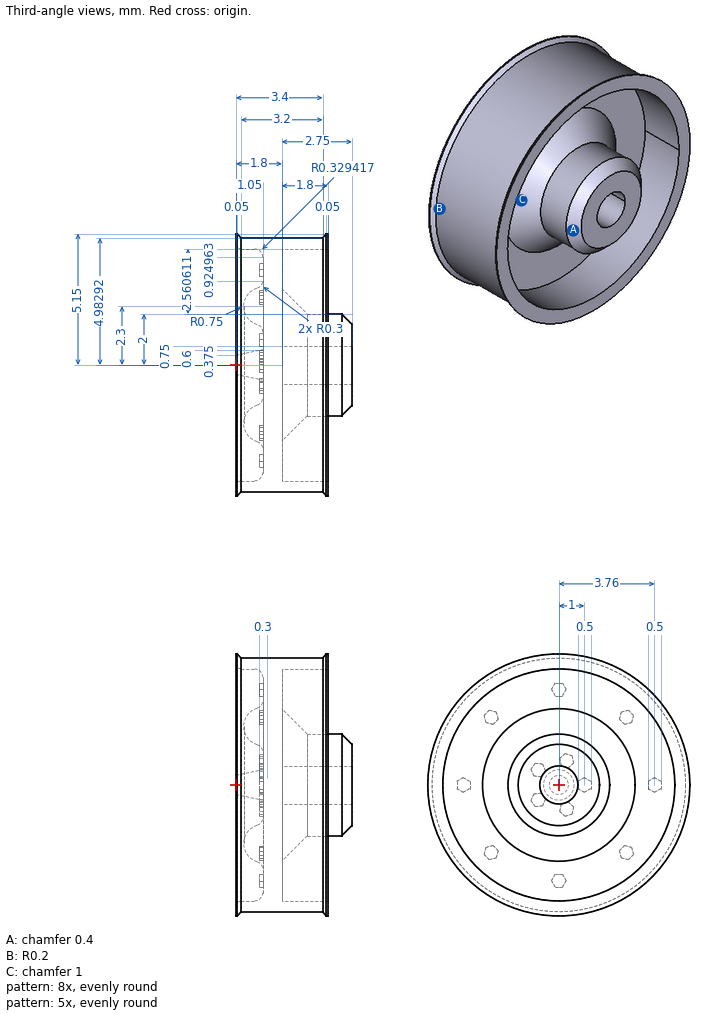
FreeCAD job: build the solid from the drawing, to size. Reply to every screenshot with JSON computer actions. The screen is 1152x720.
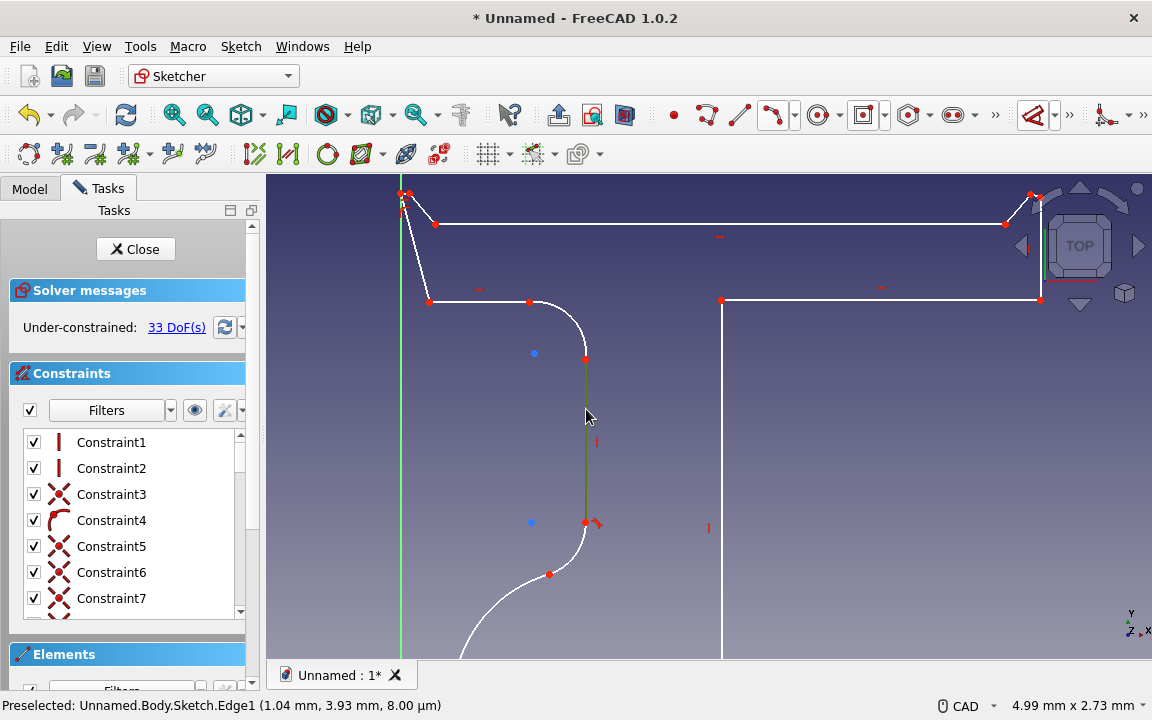
{"action": "left_click", "coordinate": [582, 333]}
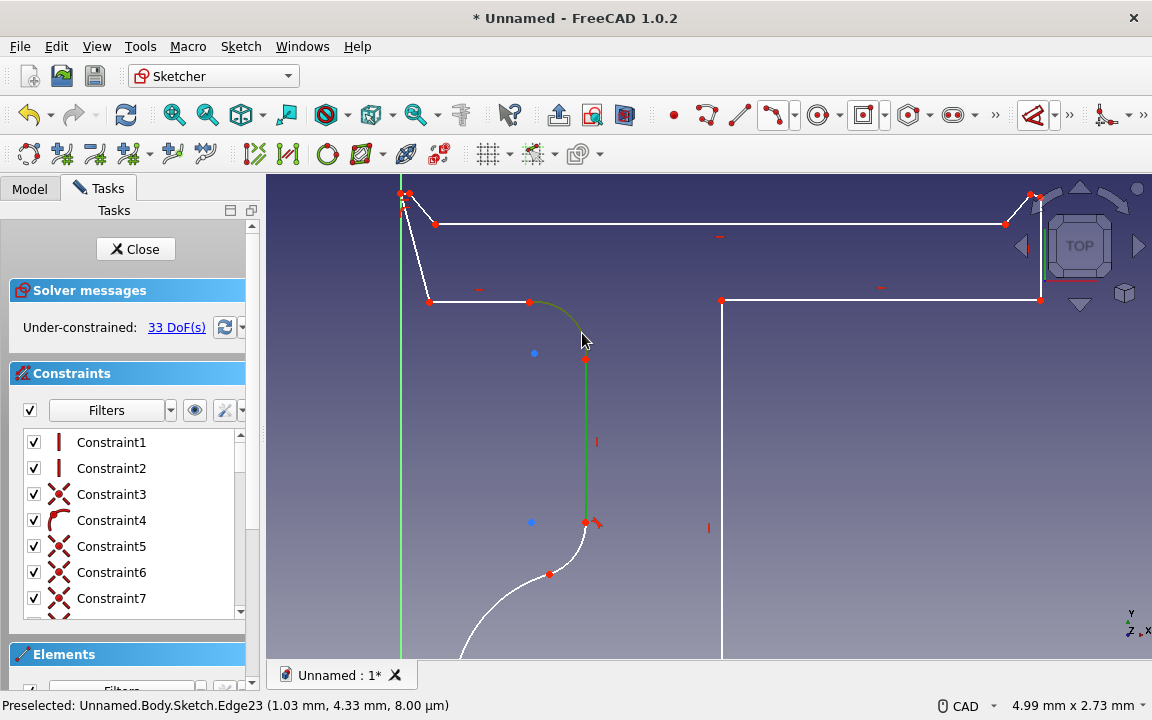
{"action": "key", "text": "t"}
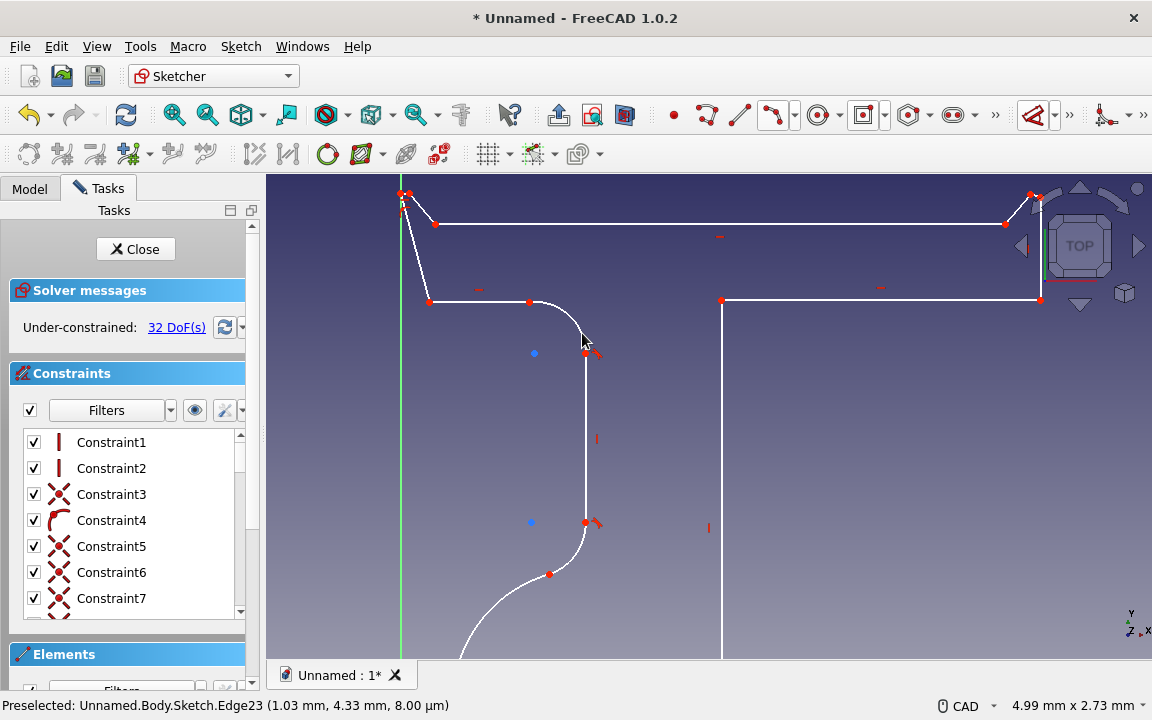
{"action": "scroll", "coordinate": [570, 316], "scroll_direction": "down", "scroll_amount": 6}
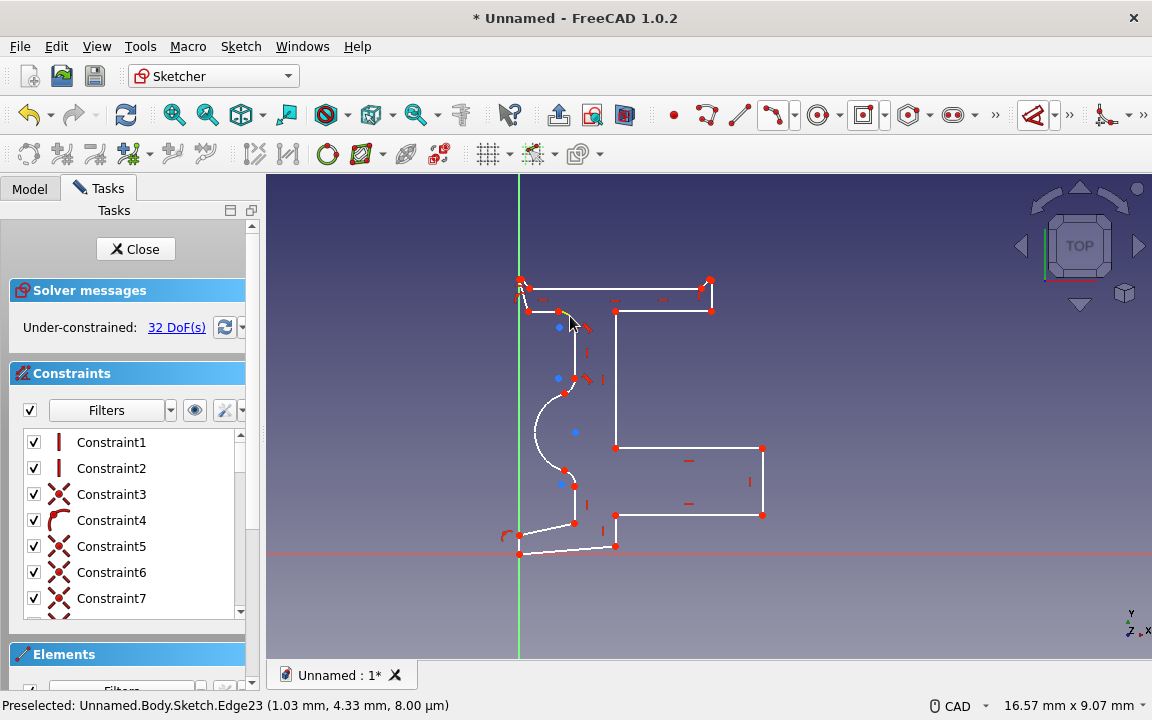
{"action": "scroll", "coordinate": [575, 498], "scroll_direction": "up", "scroll_amount": 2}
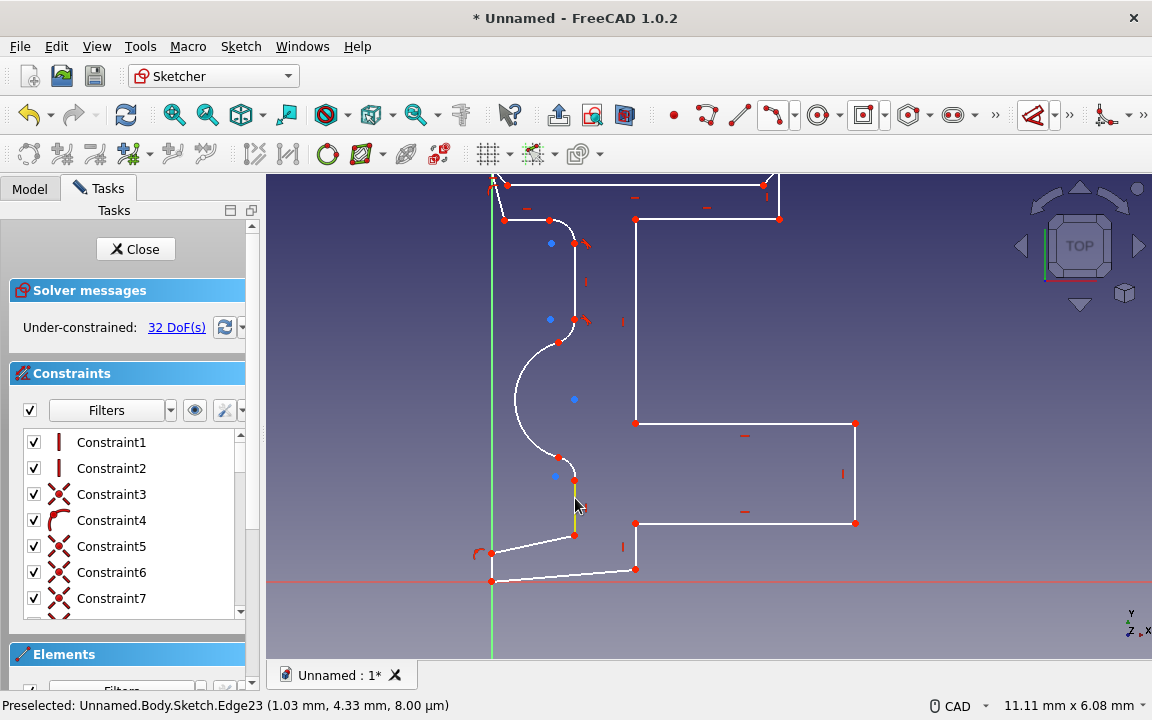
{"action": "left_click", "coordinate": [575, 497]}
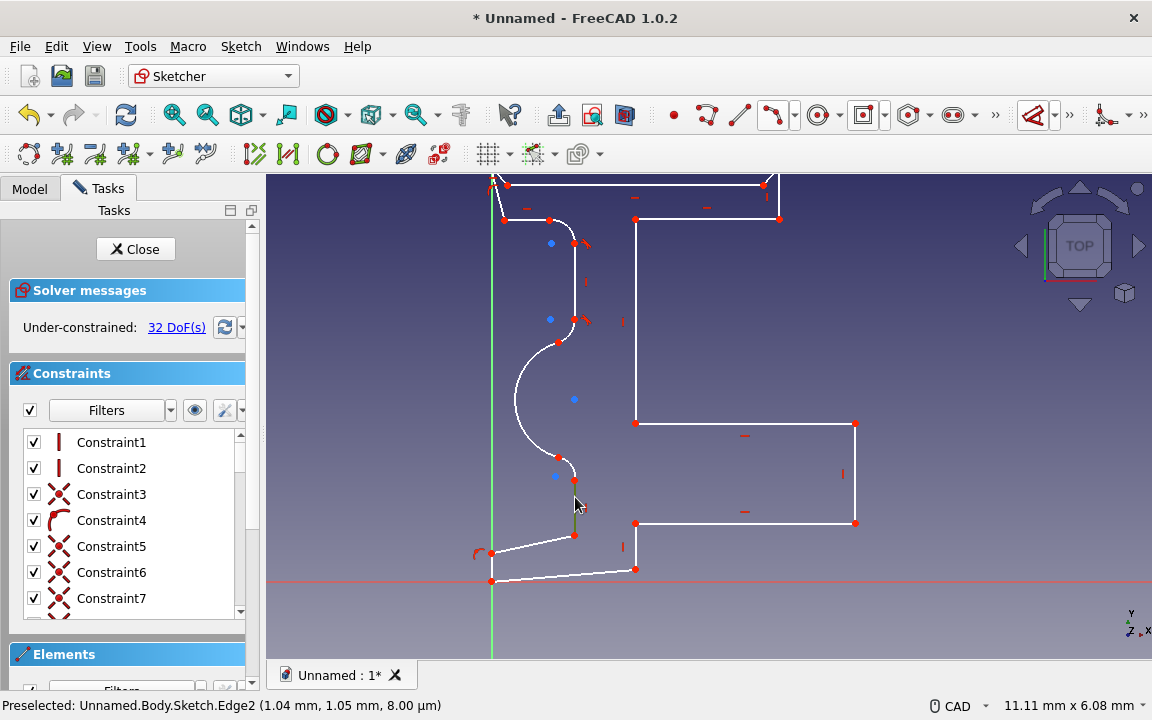
{"action": "scroll", "coordinate": [574, 471], "scroll_direction": "up", "scroll_amount": 2}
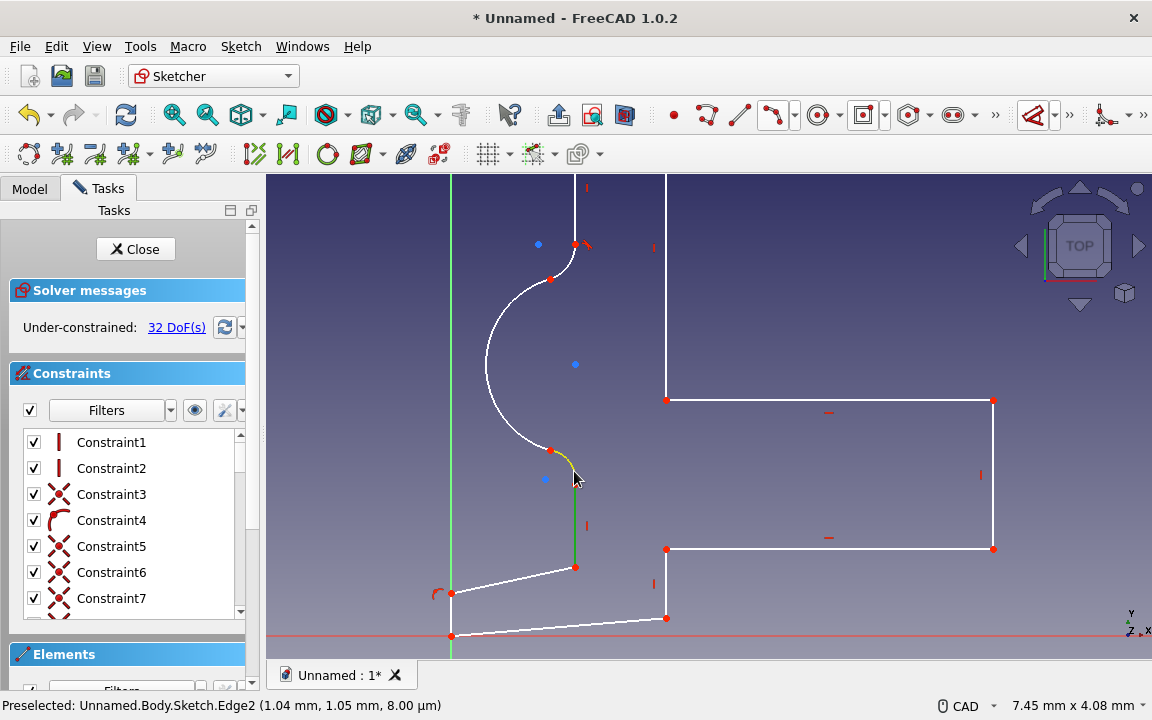
{"action": "left_click", "coordinate": [574, 471]}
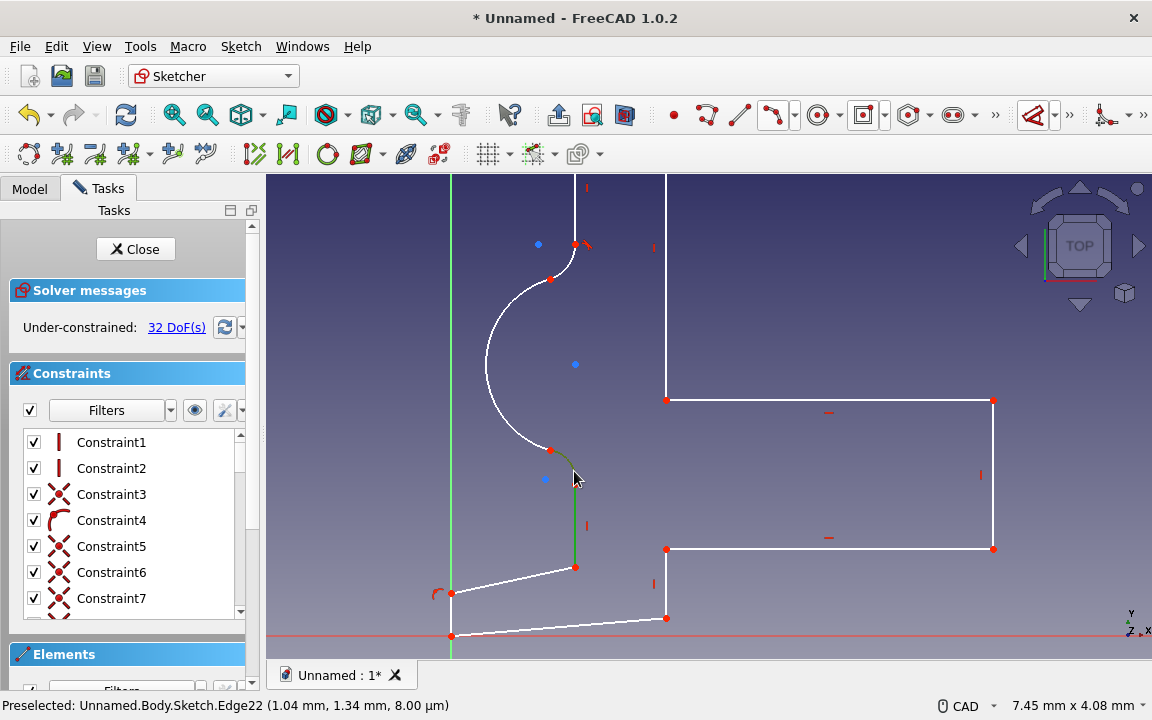
{"action": "key", "text": "t"}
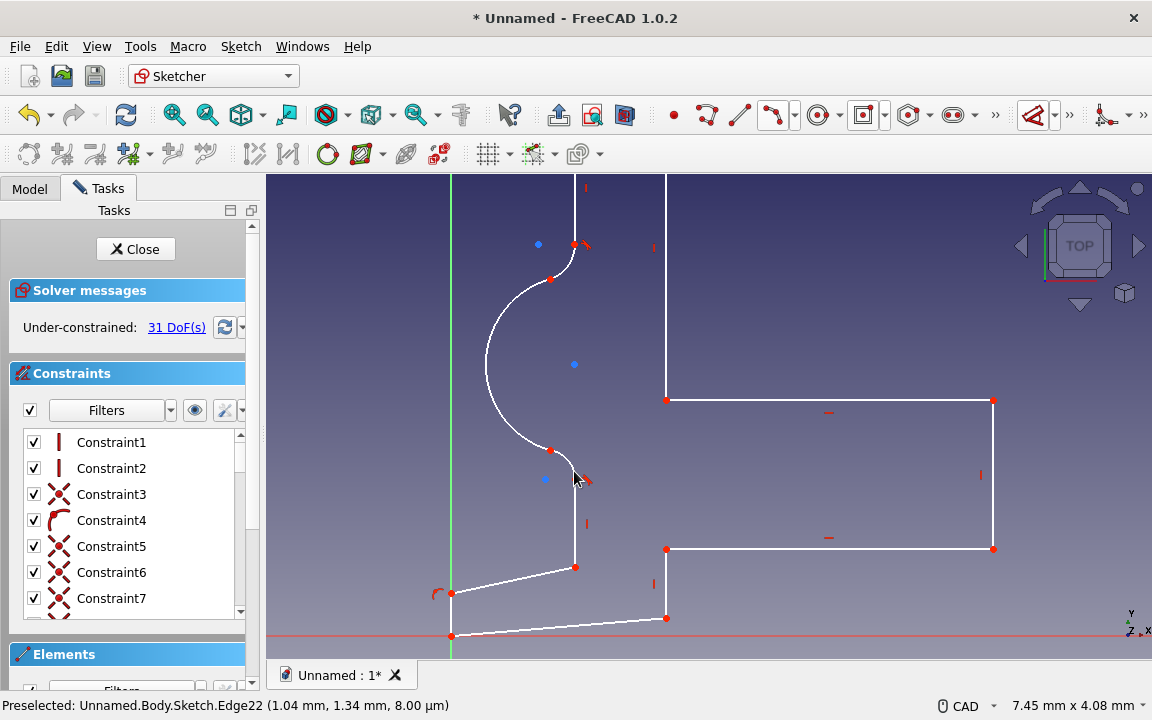
{"action": "scroll", "coordinate": [574, 487], "scroll_direction": "down", "scroll_amount": 4}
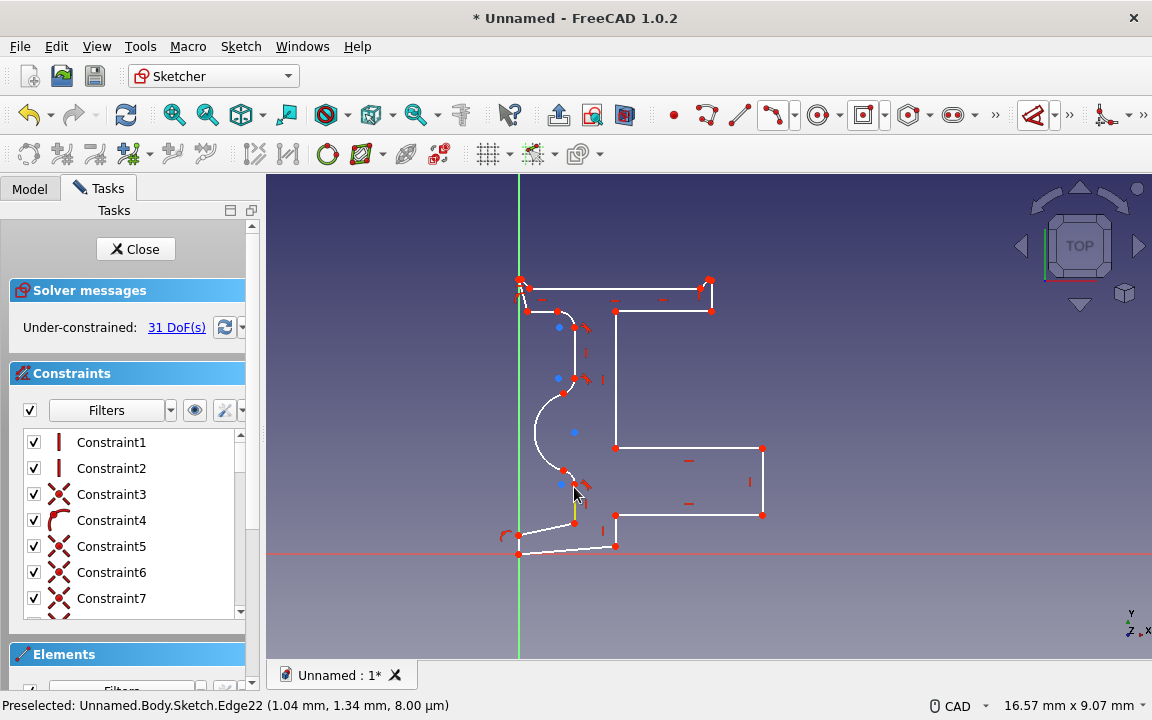
{"action": "scroll", "coordinate": [537, 312], "scroll_direction": "up", "scroll_amount": 3}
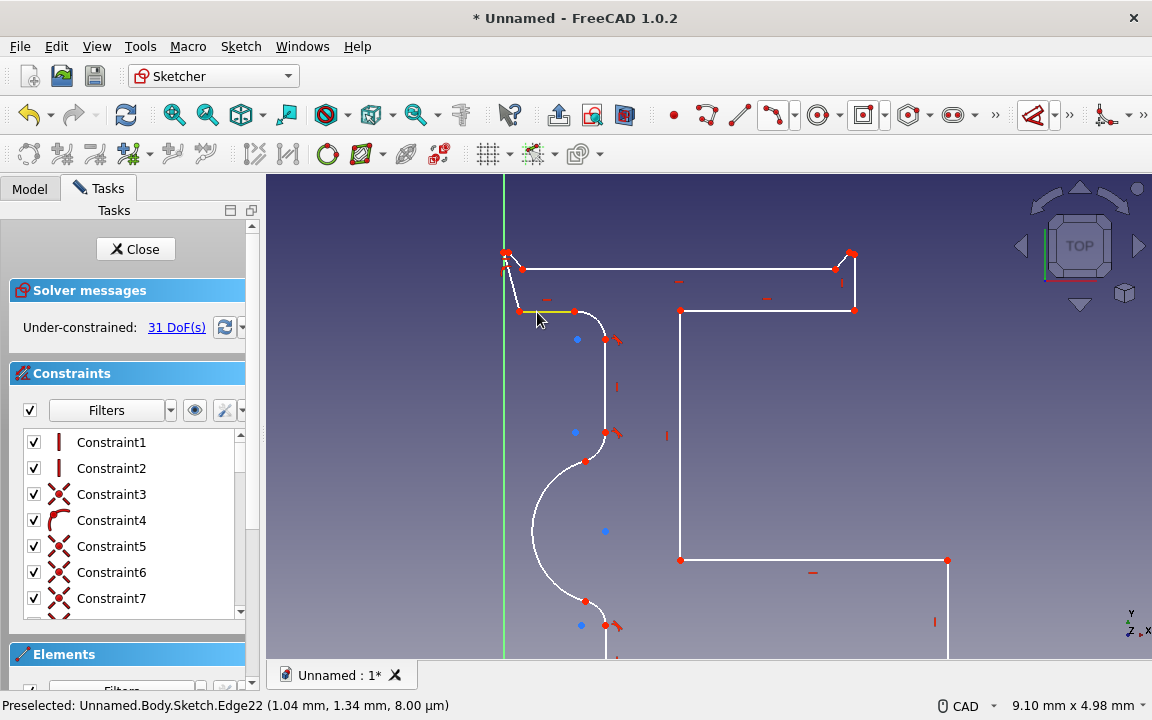
{"action": "left_click", "coordinate": [536, 312]}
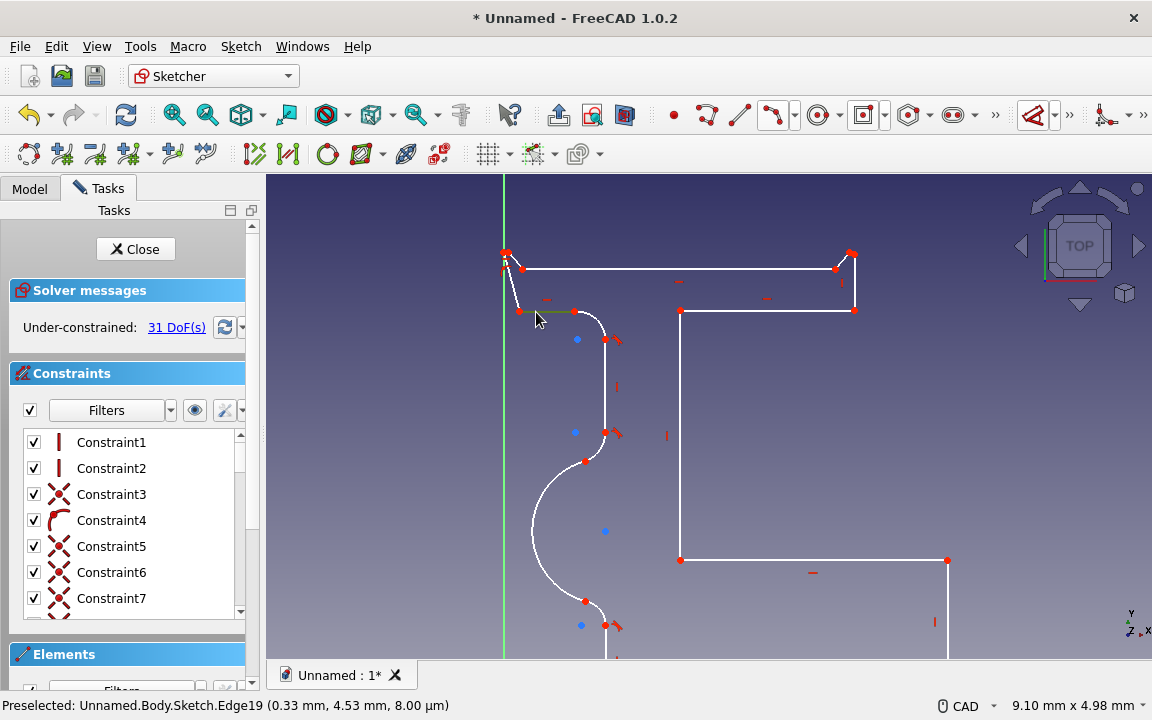
{"action": "left_click", "coordinate": [602, 326]}